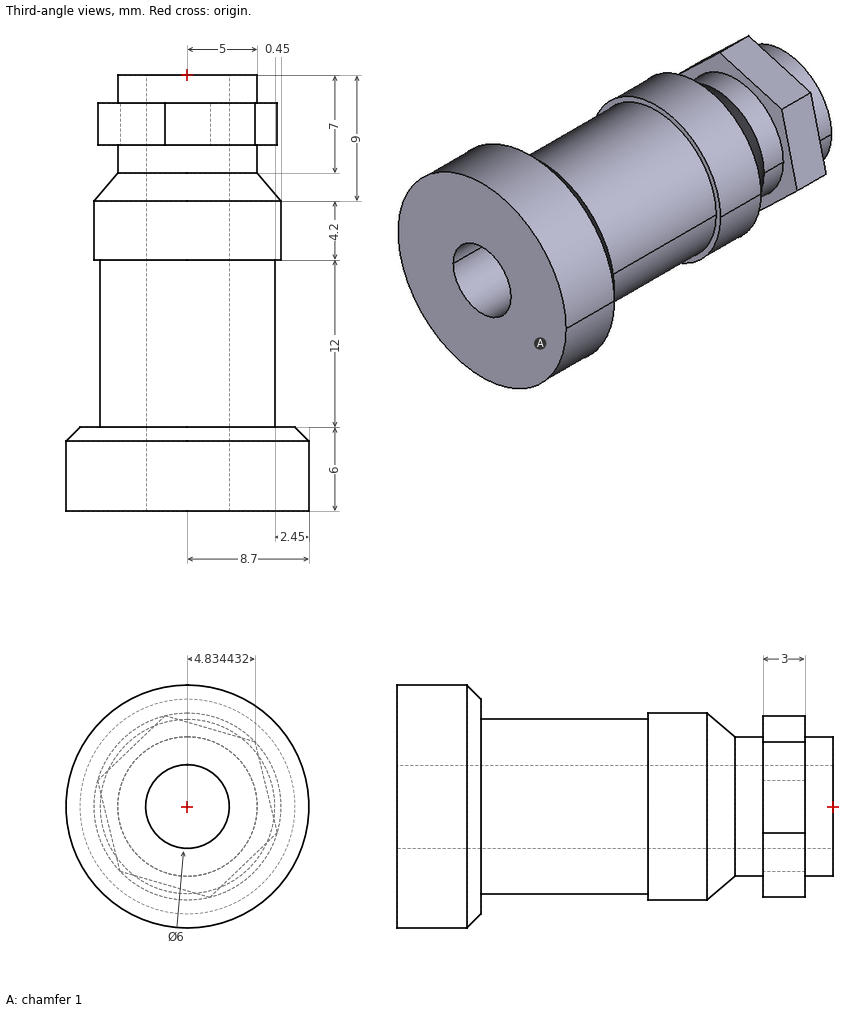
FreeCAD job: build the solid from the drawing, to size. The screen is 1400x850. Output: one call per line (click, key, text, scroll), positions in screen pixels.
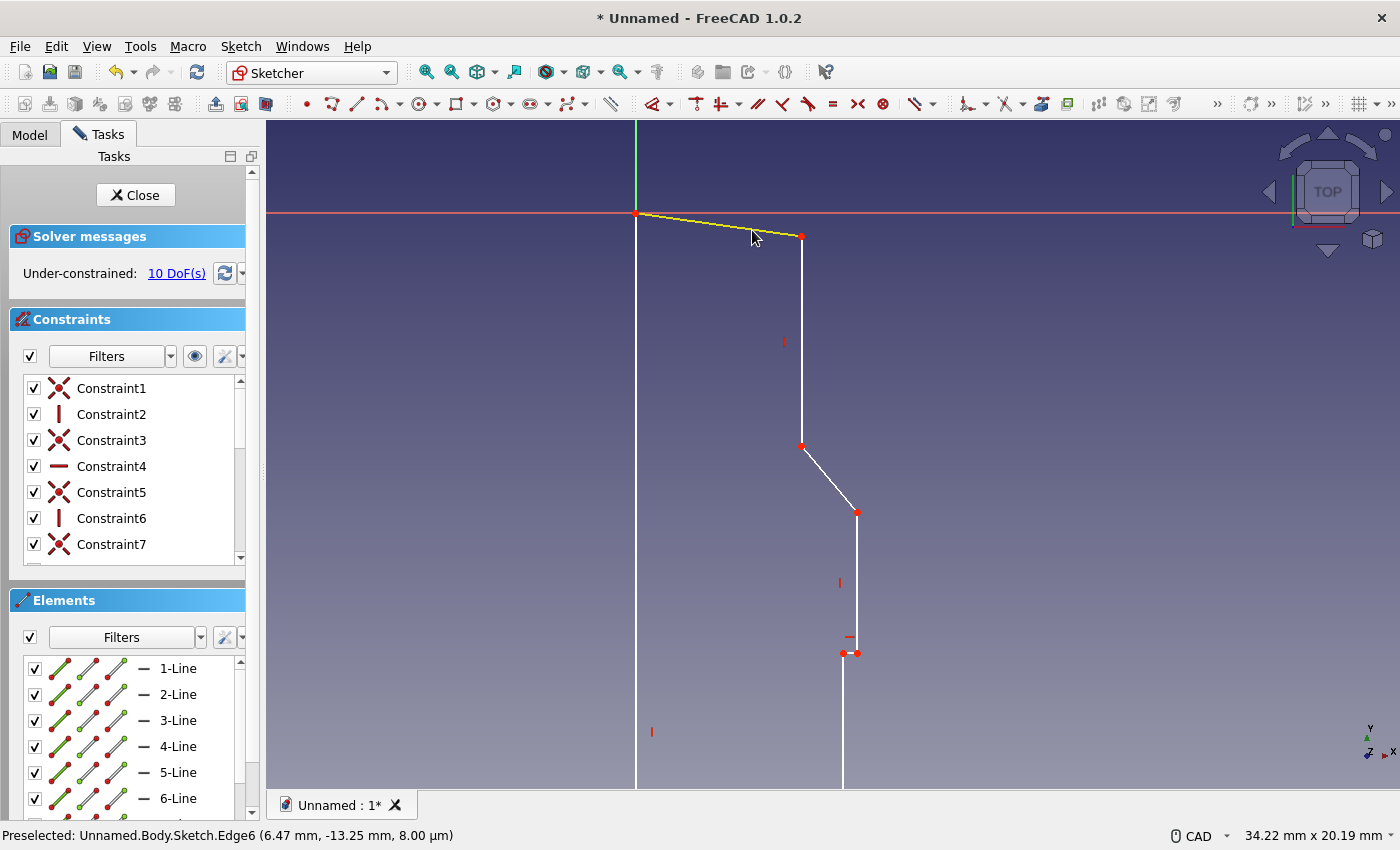
click(752, 230)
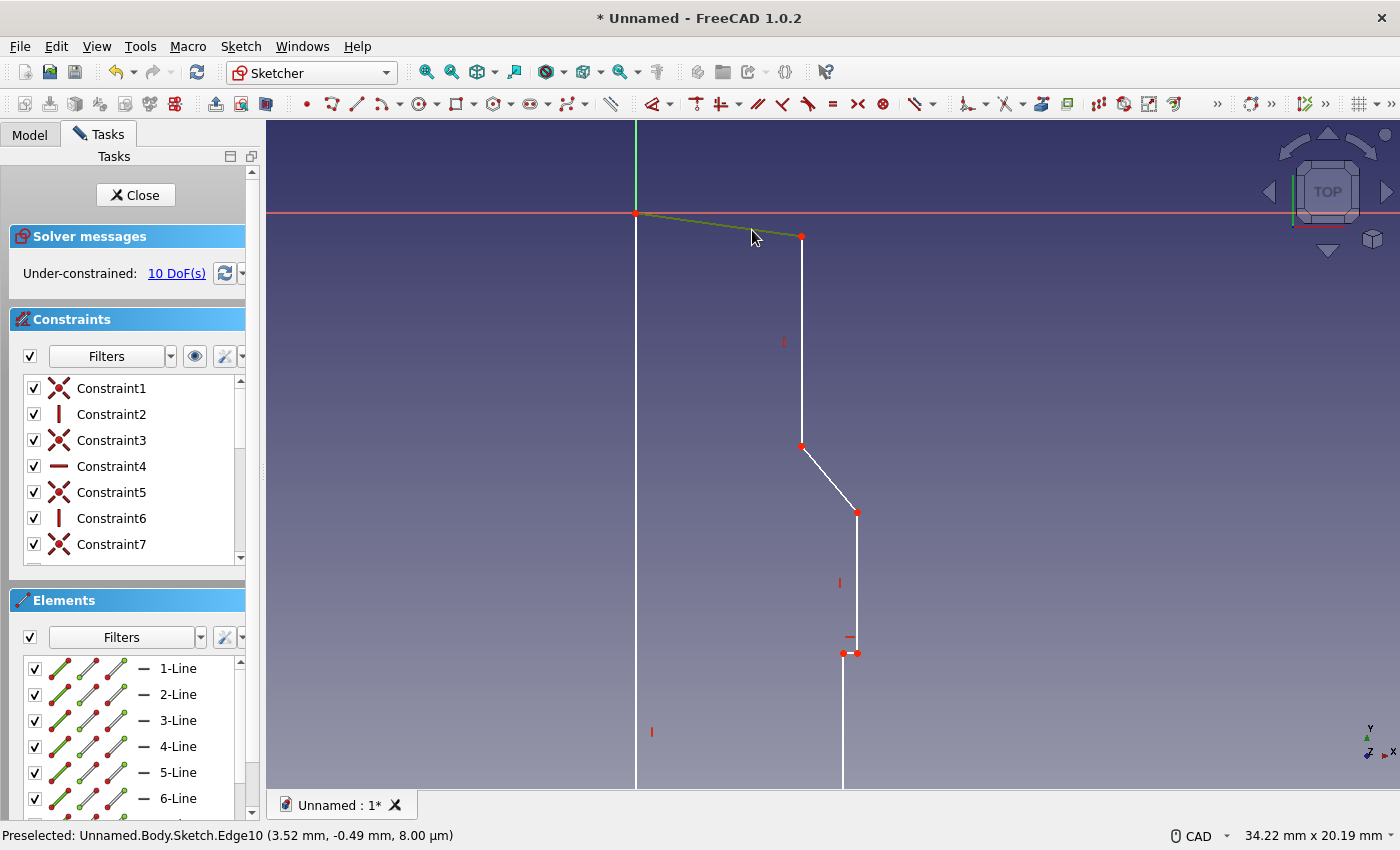
click(738, 104)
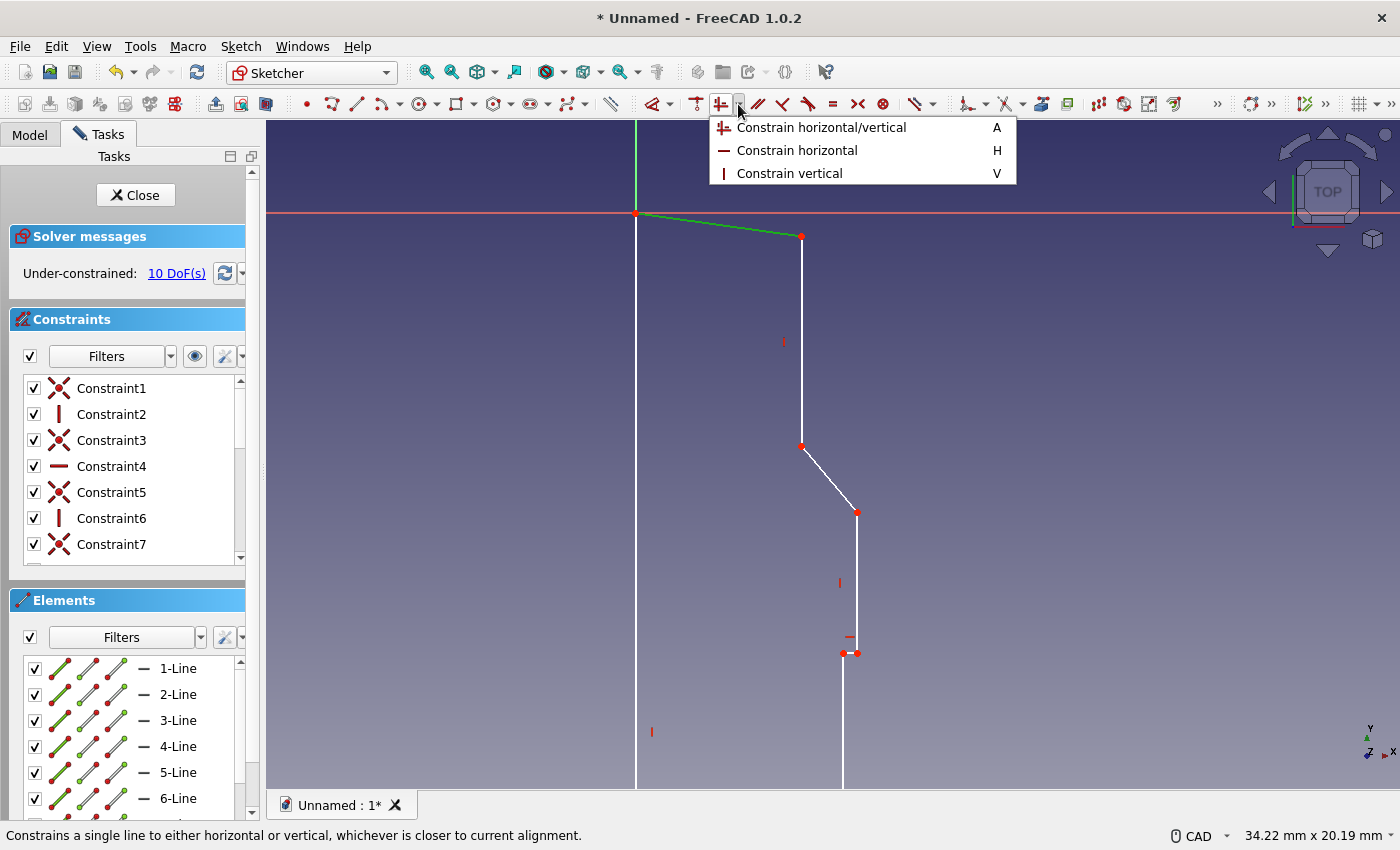
click(863, 150)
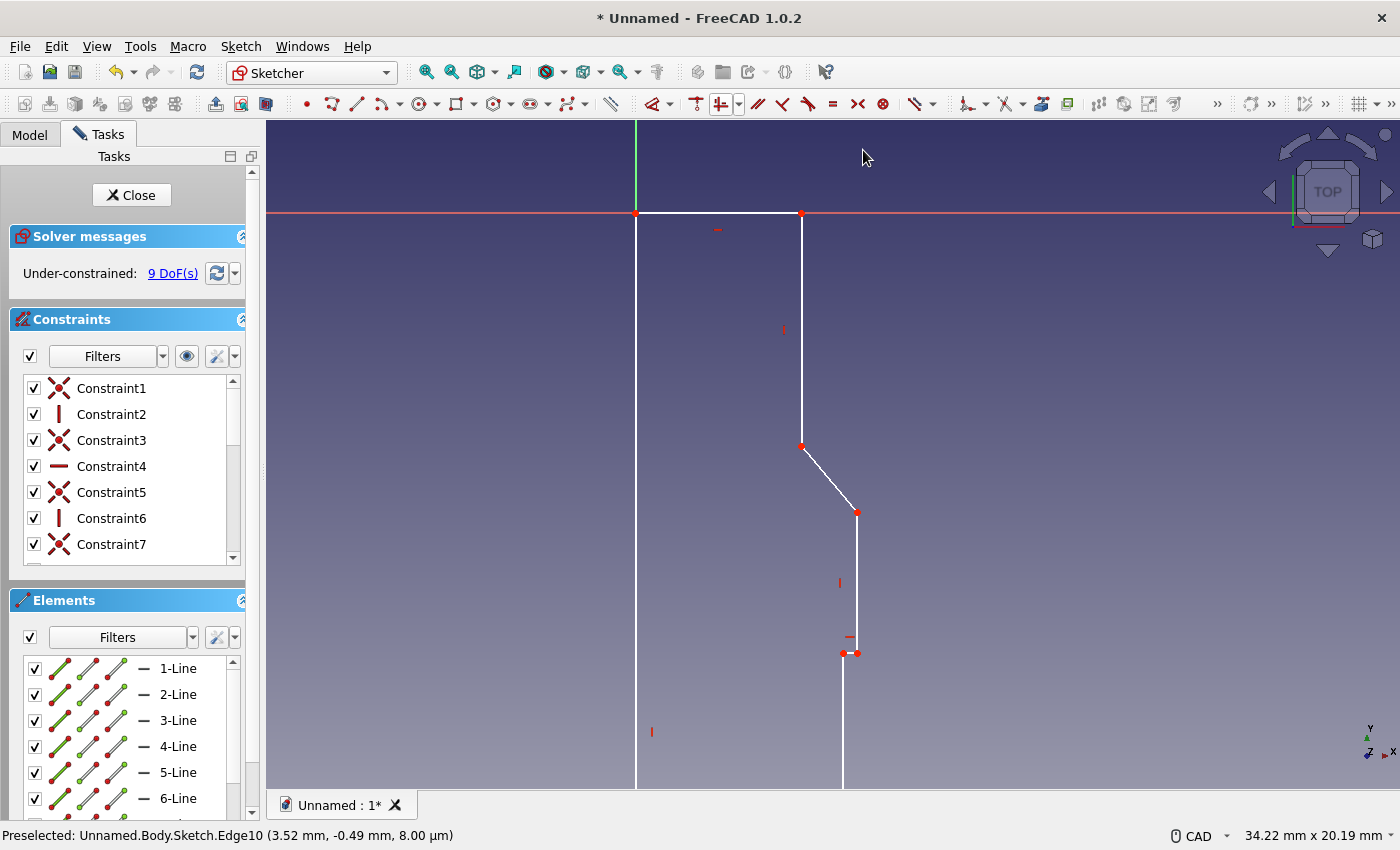
click(652, 104)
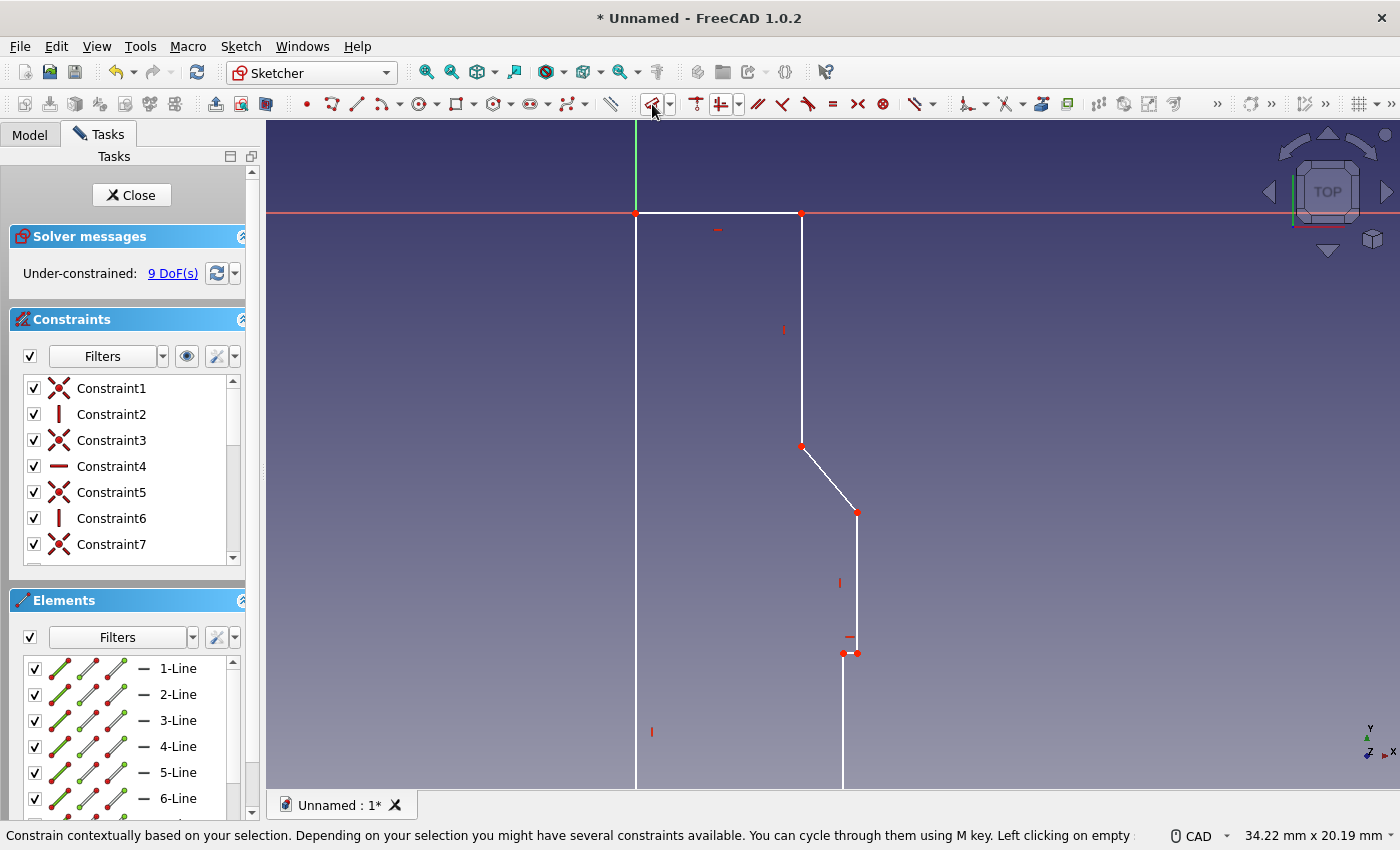
scroll(752, 230, down, 4)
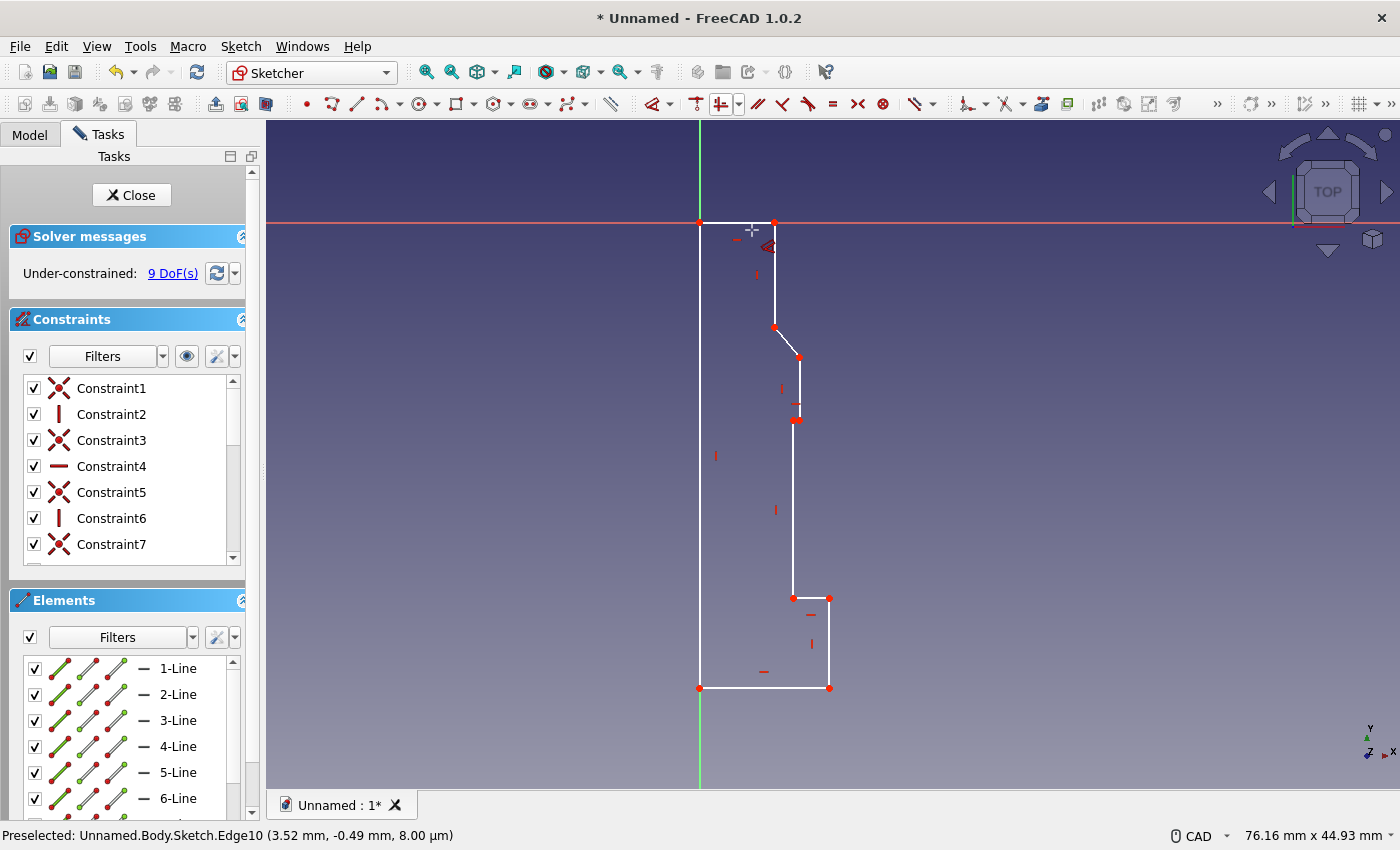
click(829, 661)
click(863, 643)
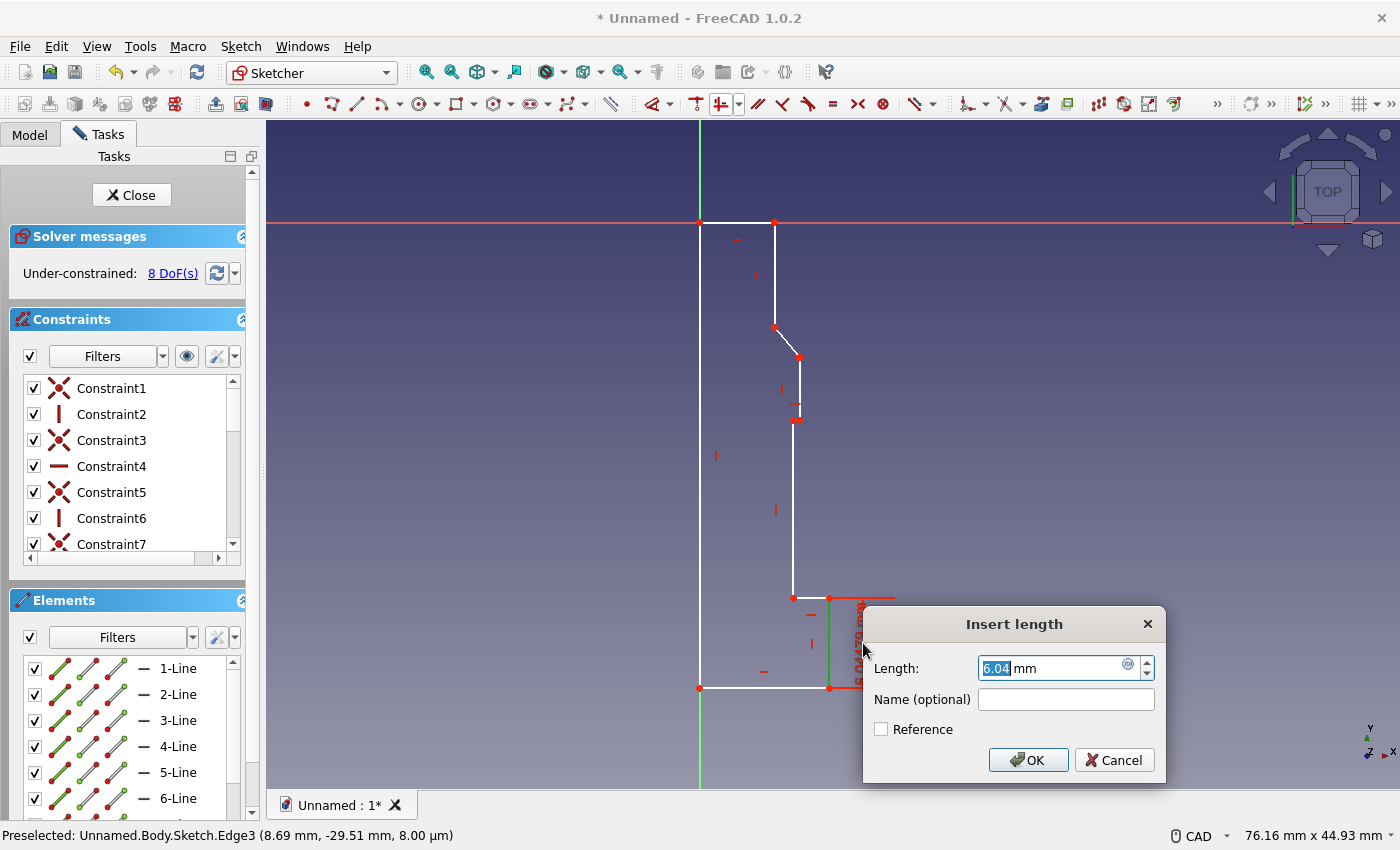
text(6)
key(Return)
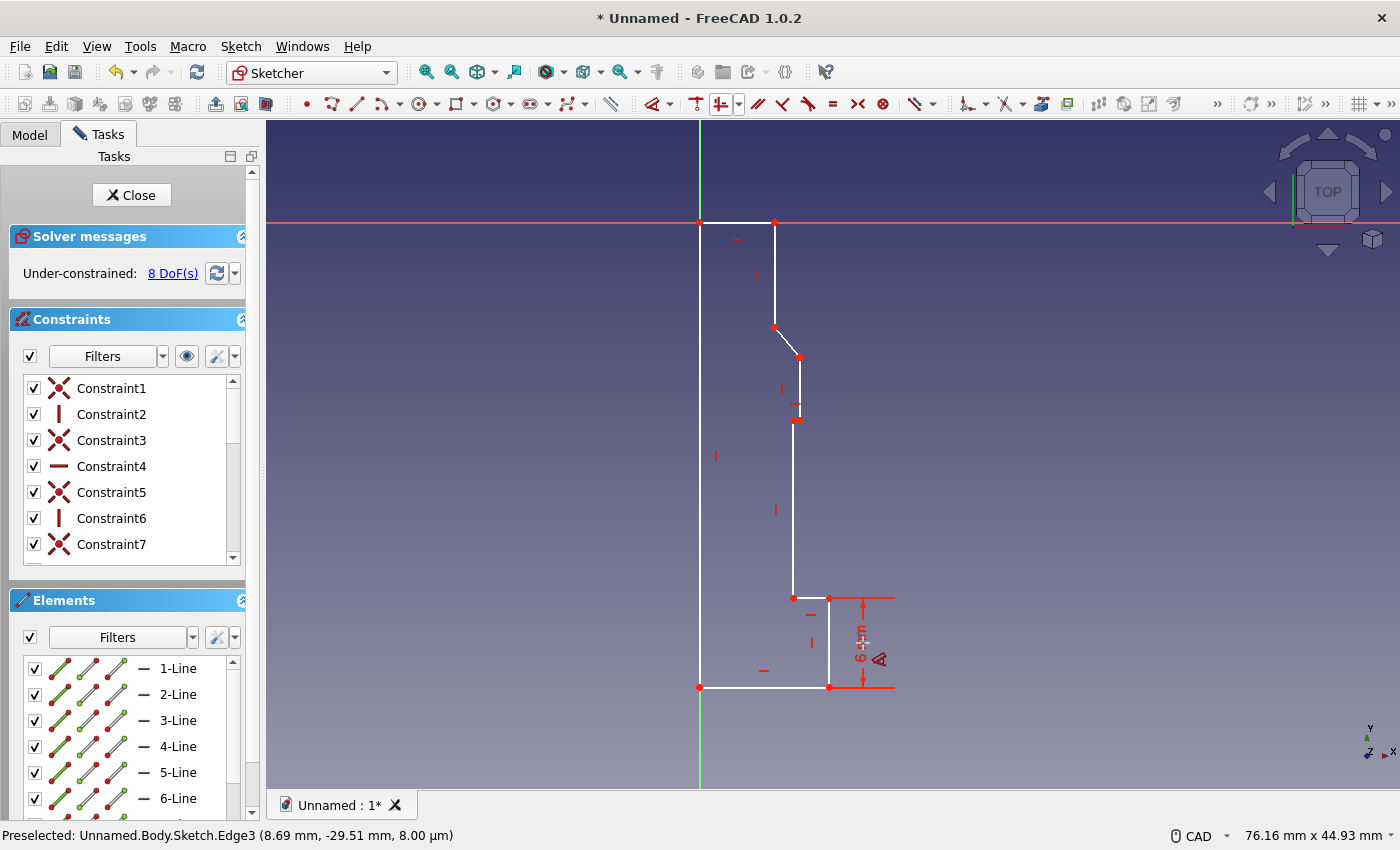
click(775, 296)
click(809, 275)